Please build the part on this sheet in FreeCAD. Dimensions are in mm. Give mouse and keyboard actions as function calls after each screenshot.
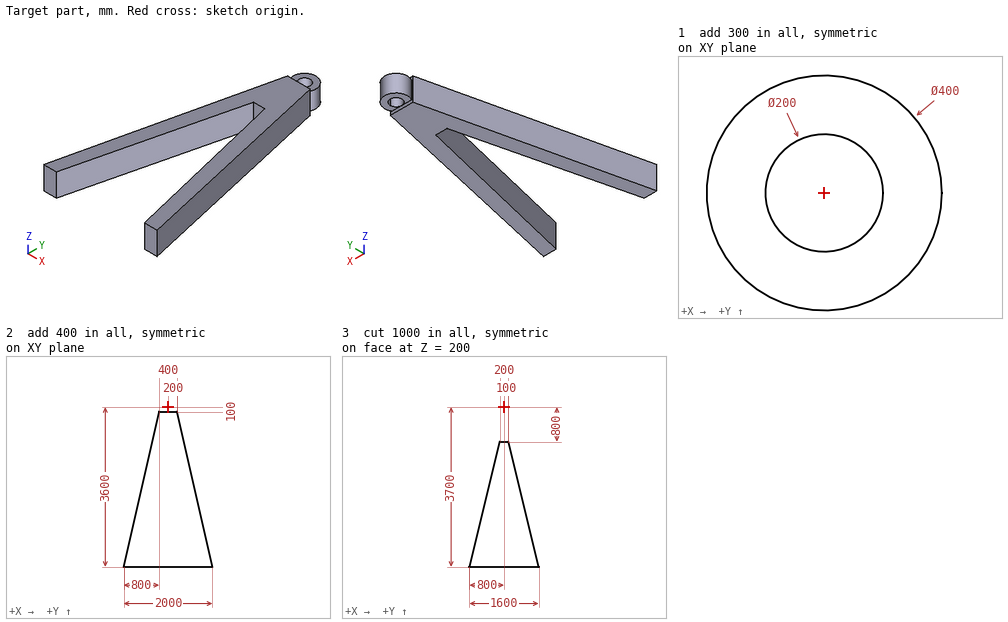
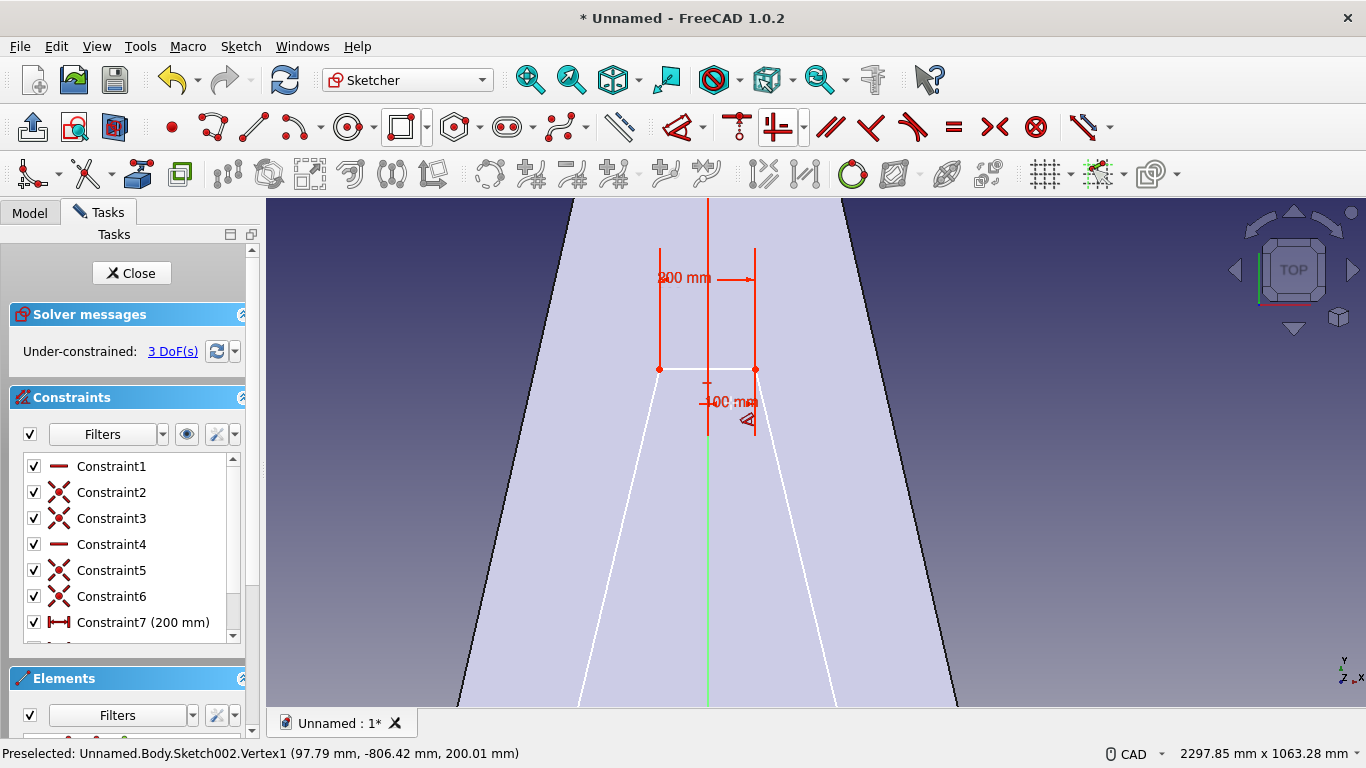
scroll(755, 370, down, 9)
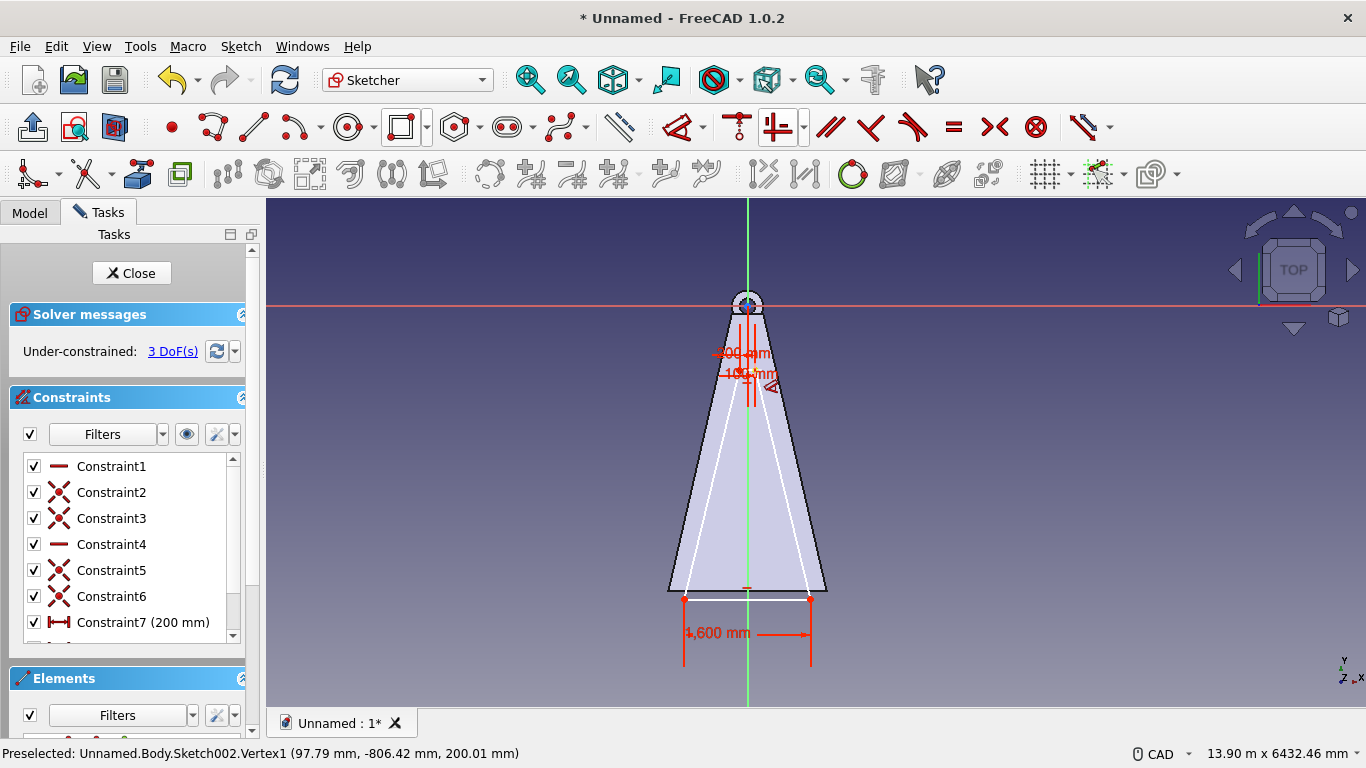
click(755, 370)
click(789, 324)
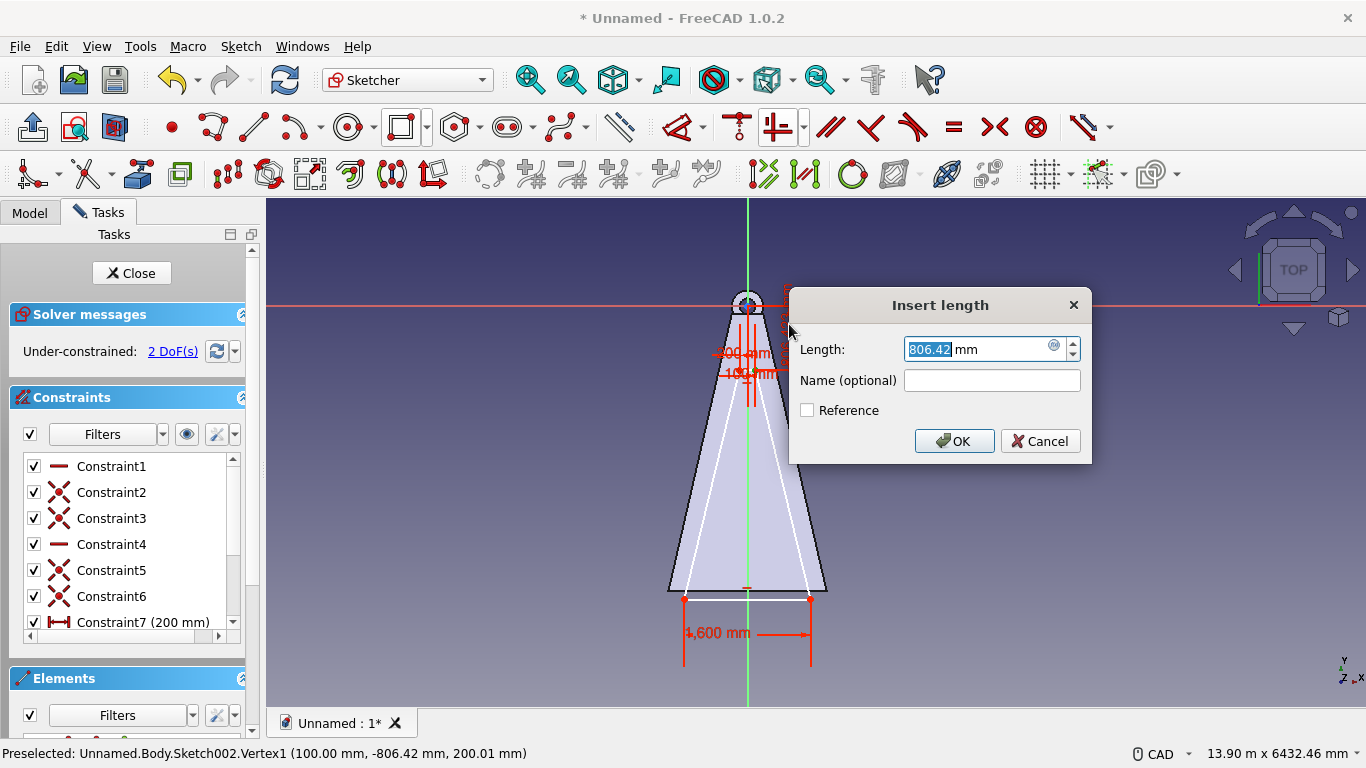
text(800)
key(Return)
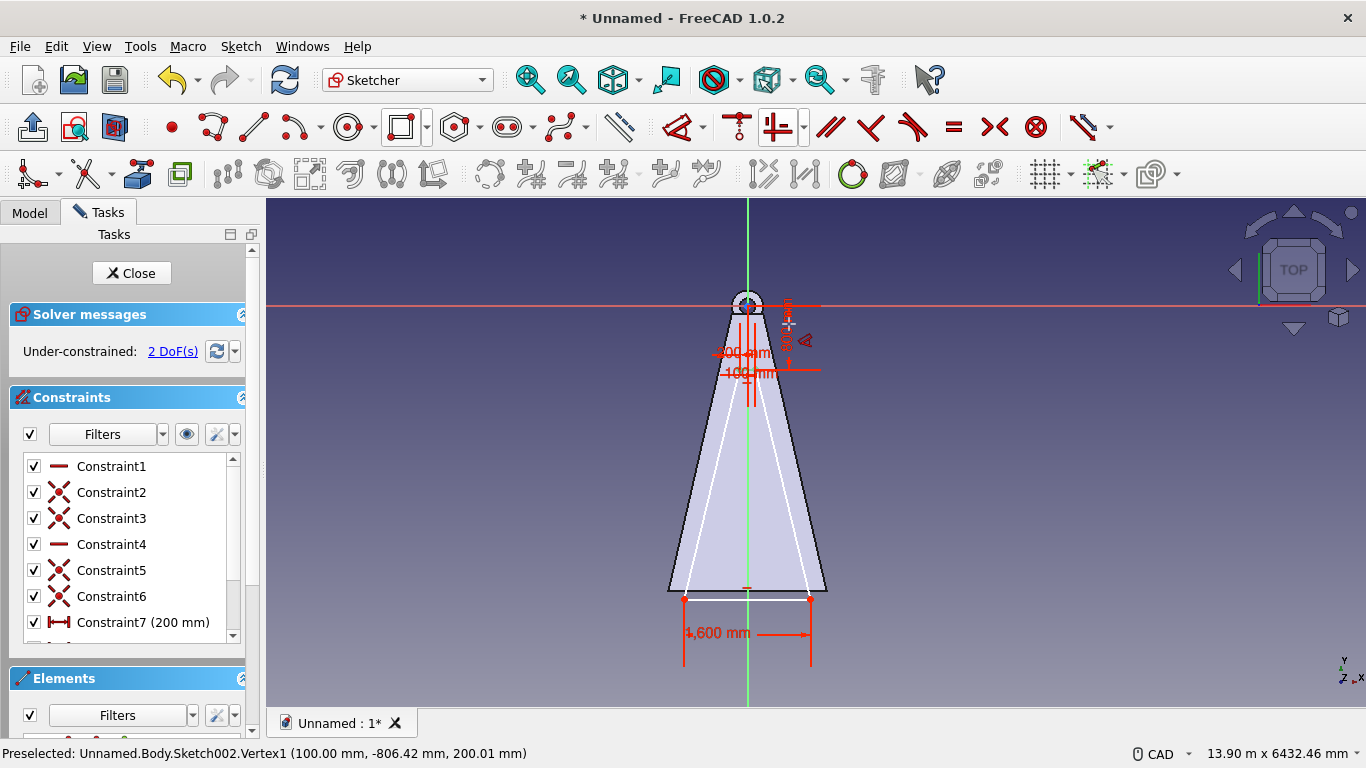
click(684, 600)
click(716, 272)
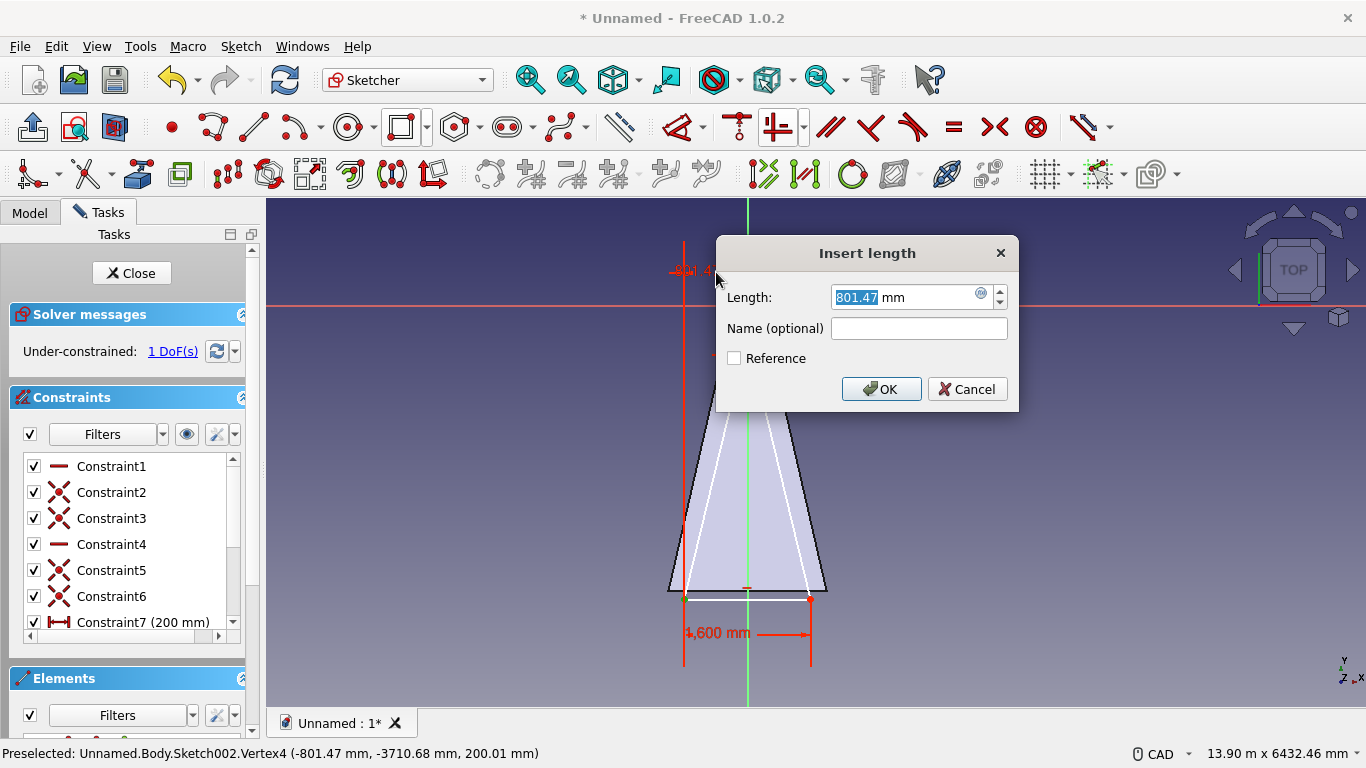
text(800)
key(Return)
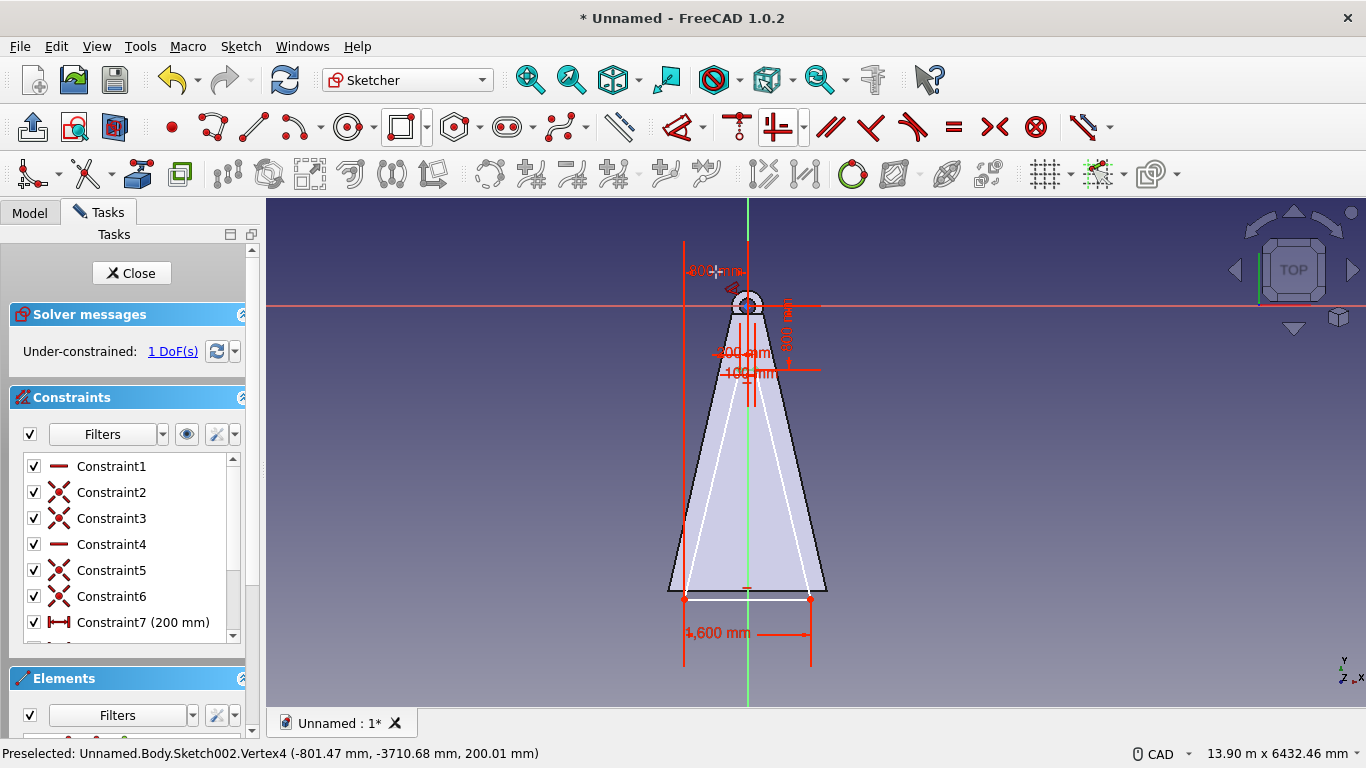
click(684, 600)
click(650, 453)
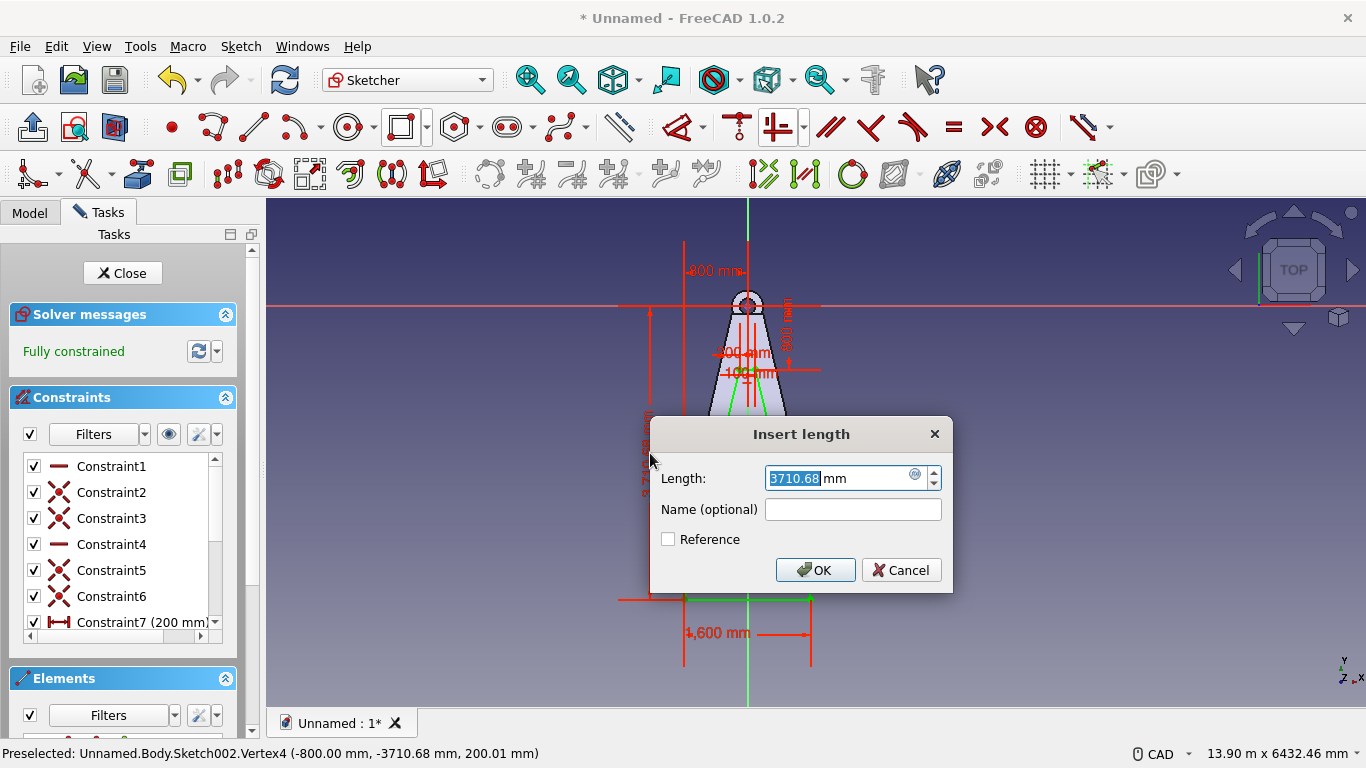
text(3700)
key(Return)
key(Escape)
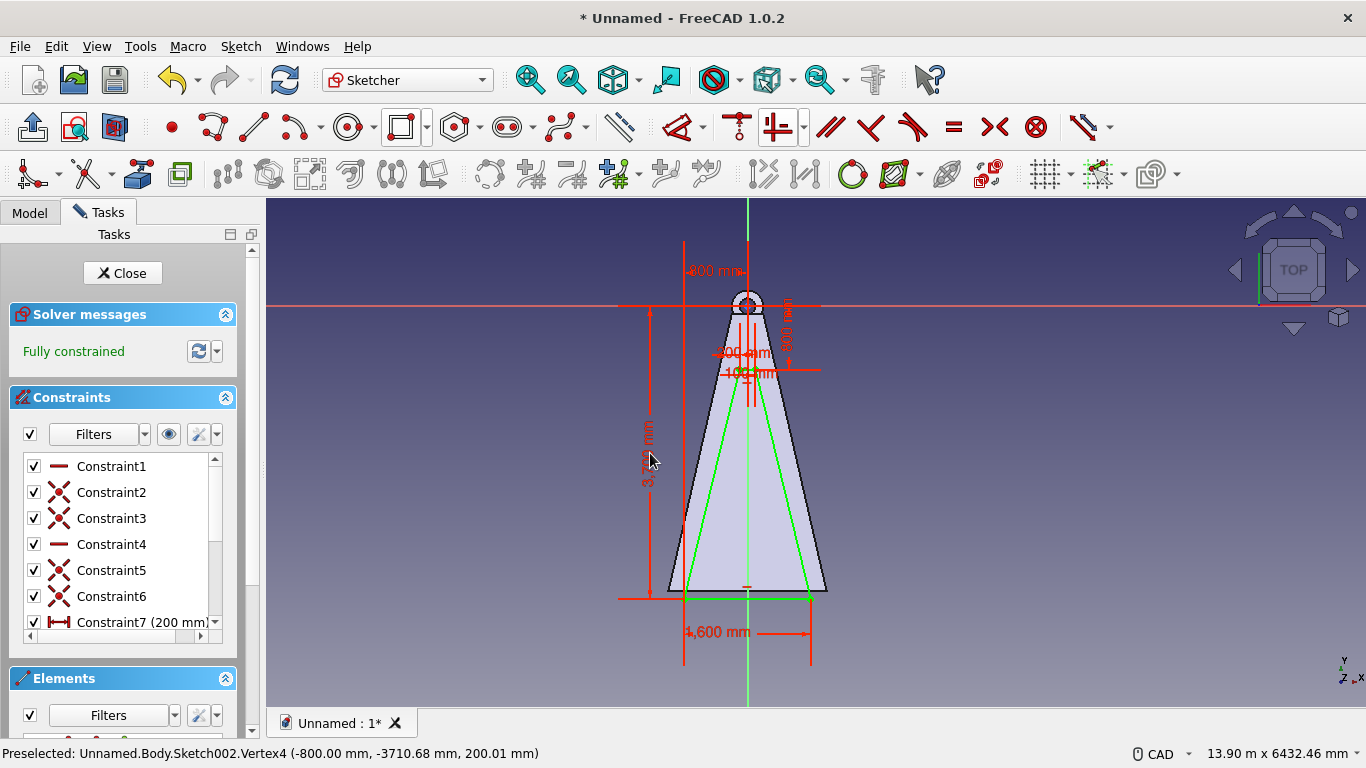
click(123, 273)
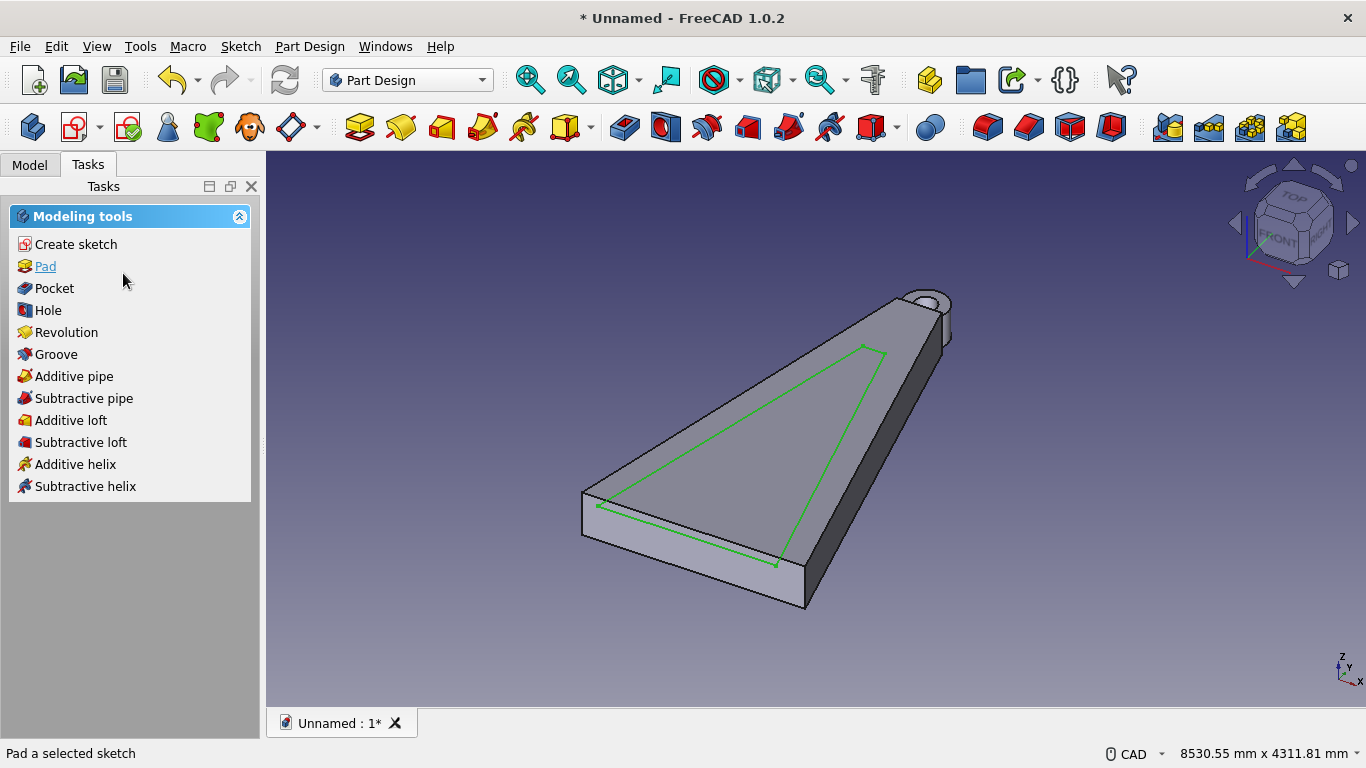
click(625, 128)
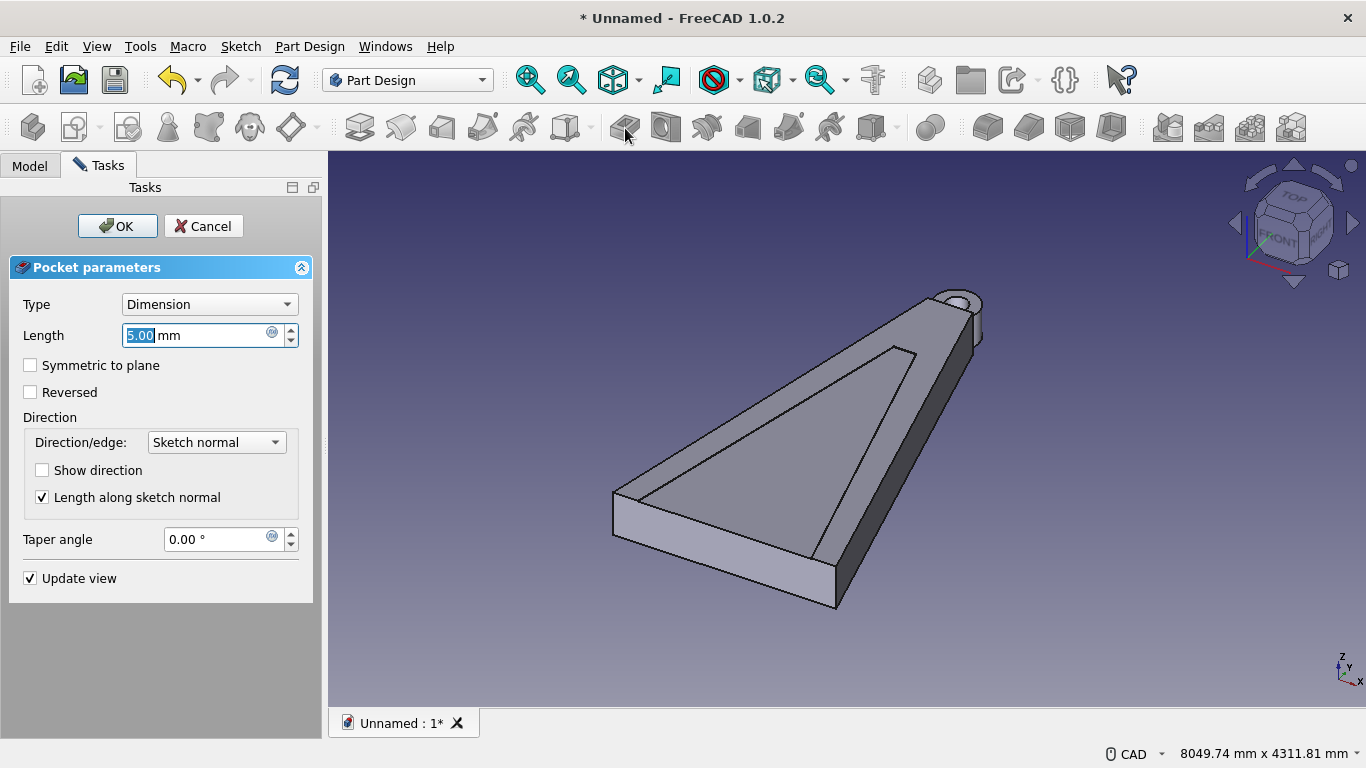
text(1000)
key(Tab)